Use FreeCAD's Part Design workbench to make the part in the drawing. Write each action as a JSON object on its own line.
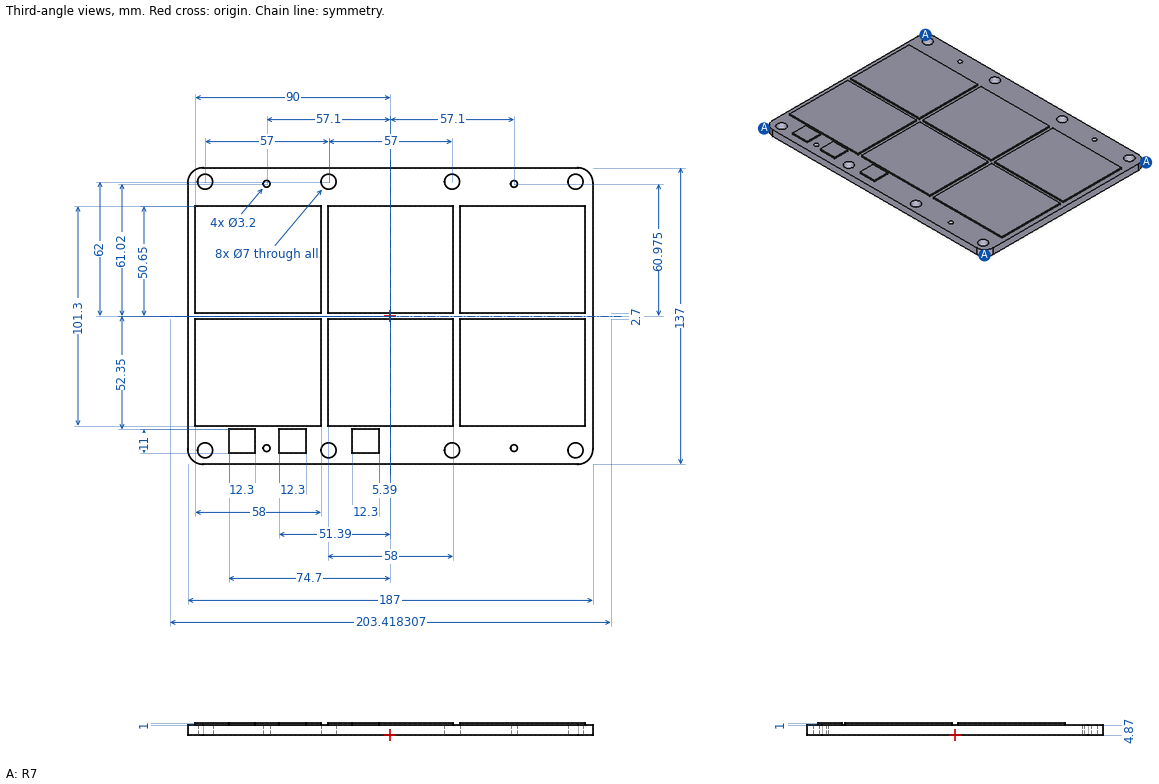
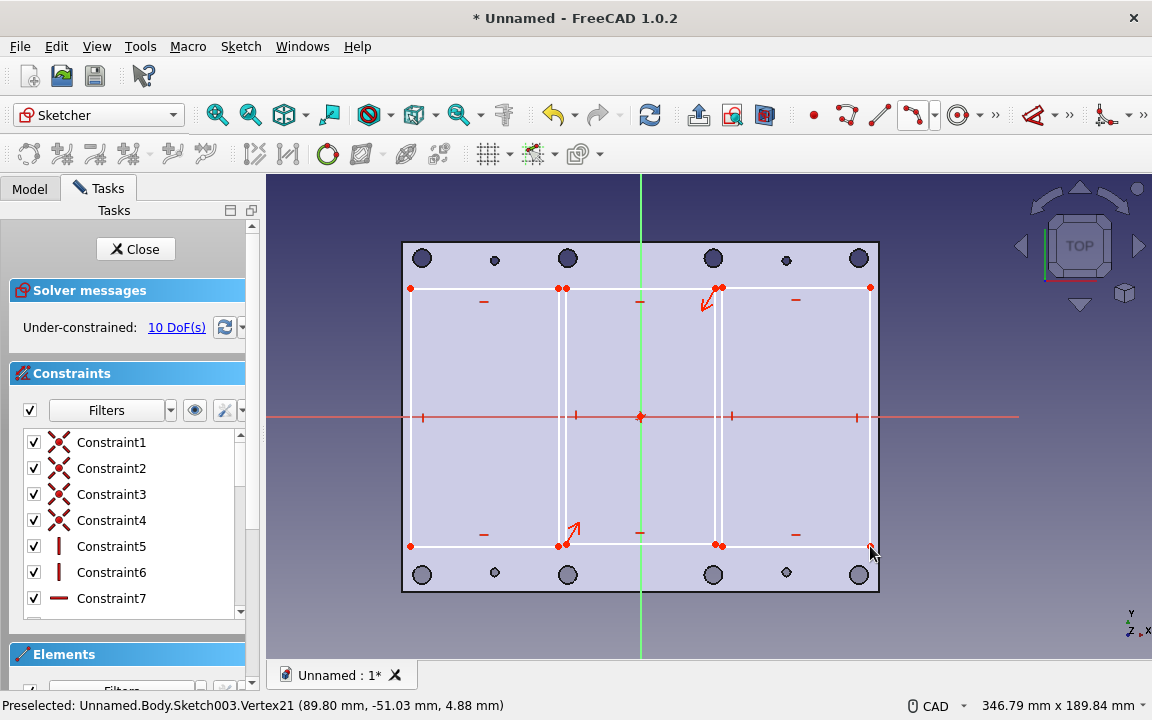
{"action": "scroll", "coordinate": [559, 289], "scroll_direction": "up", "scroll_amount": 3}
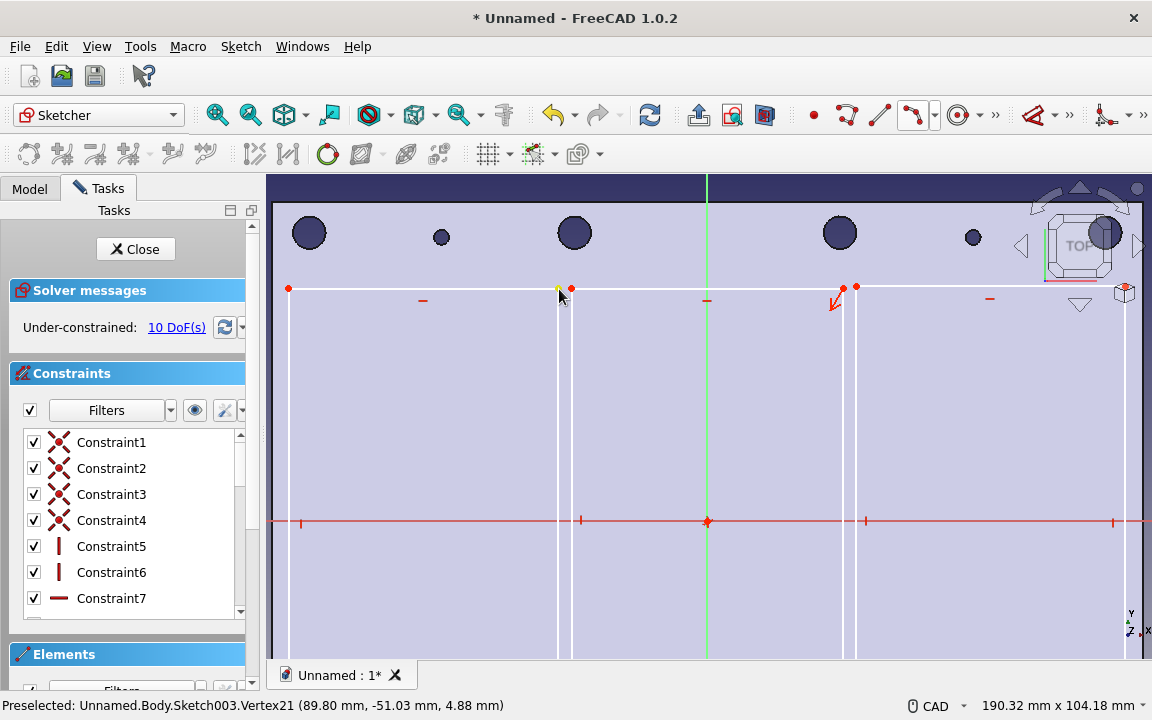
{"action": "left_click", "coordinate": [558, 289]}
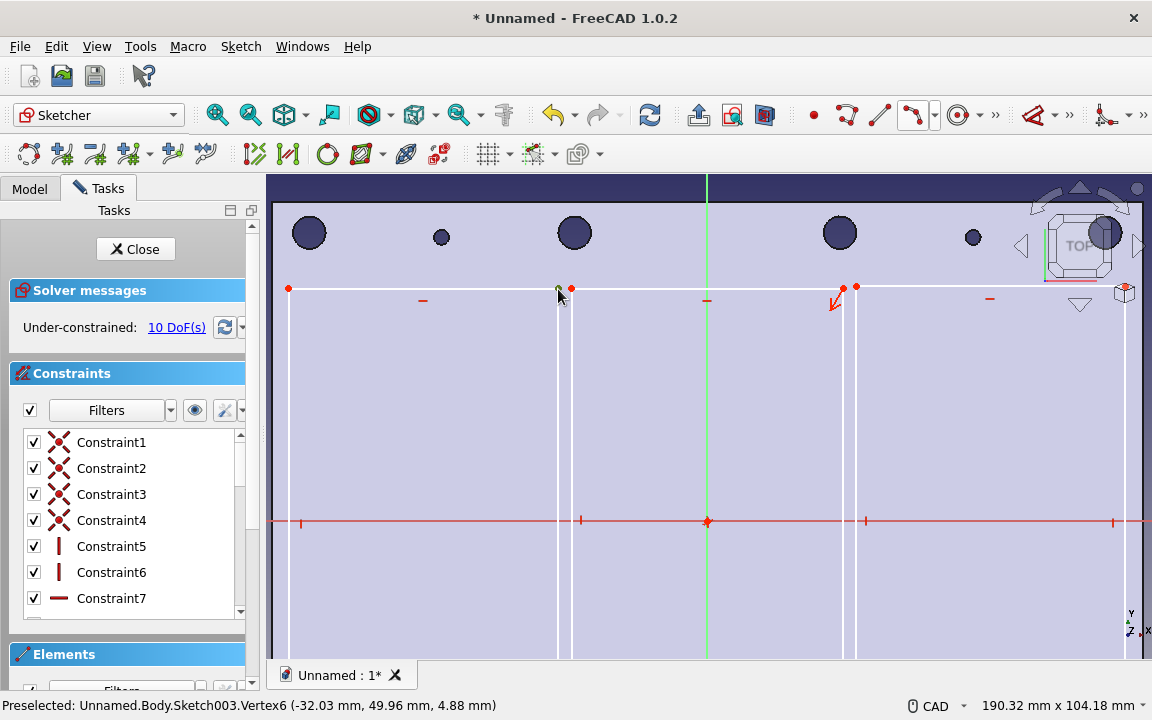
{"action": "left_click", "coordinate": [856, 286]}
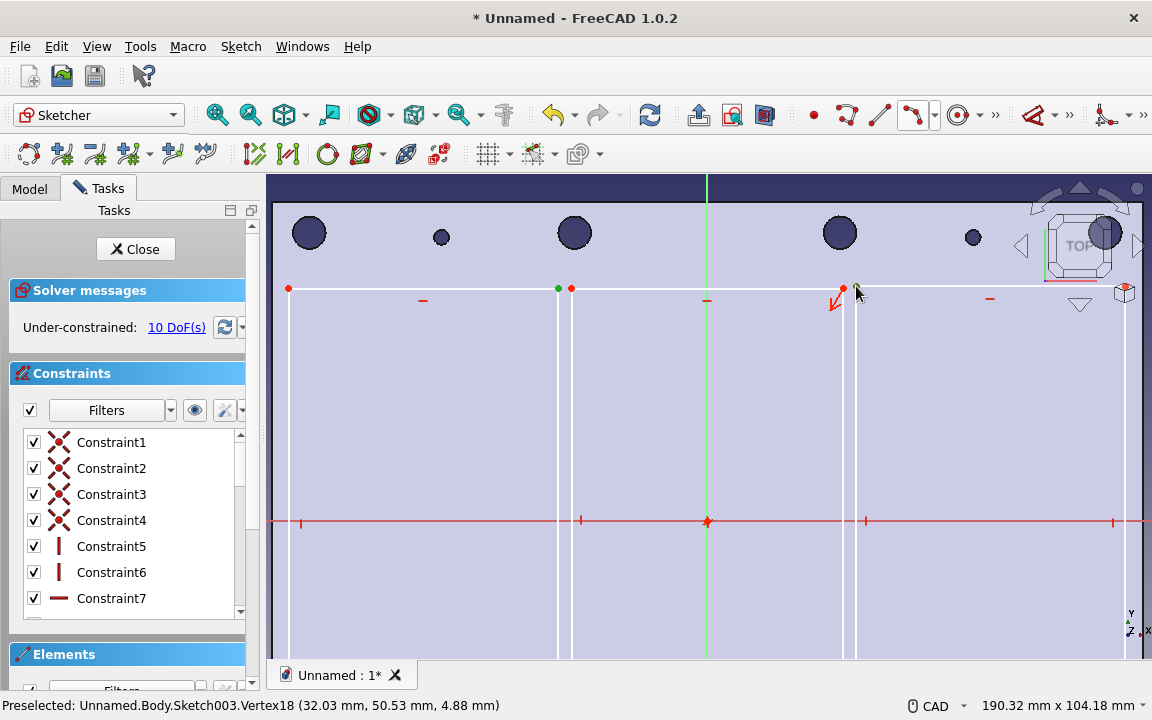
{"action": "left_click", "coordinate": [707, 600]}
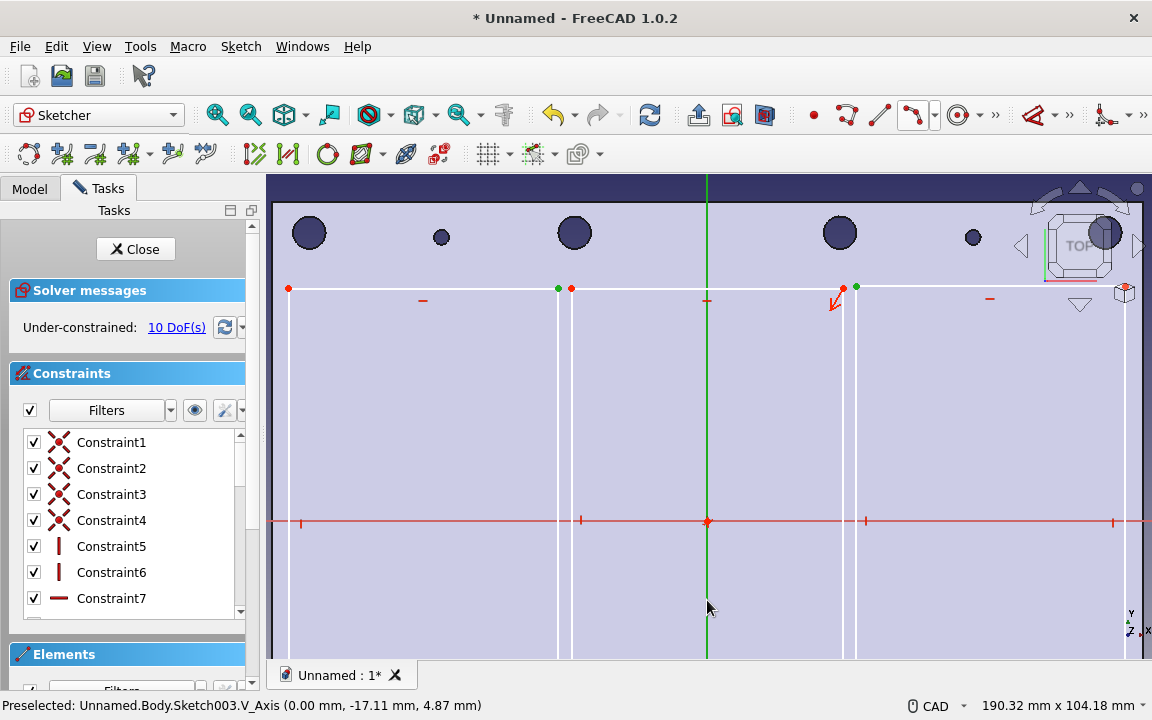
{"action": "key", "text": "s"}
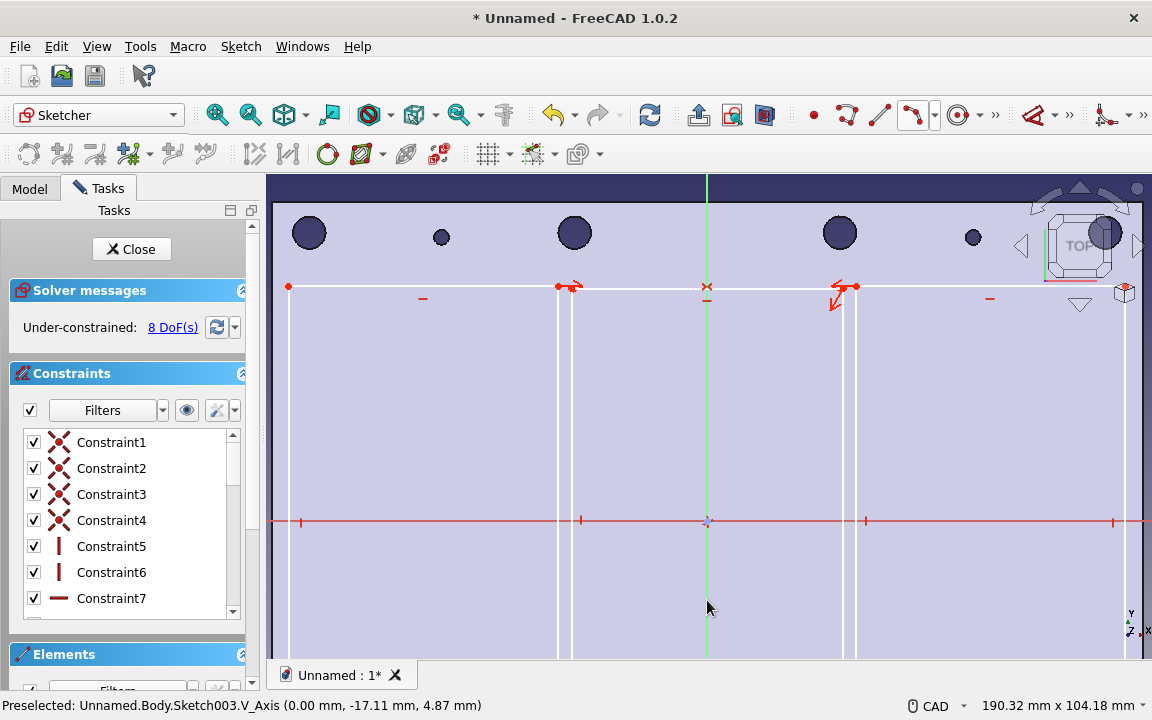
{"action": "scroll", "coordinate": [559, 289], "scroll_direction": "down", "scroll_amount": 3}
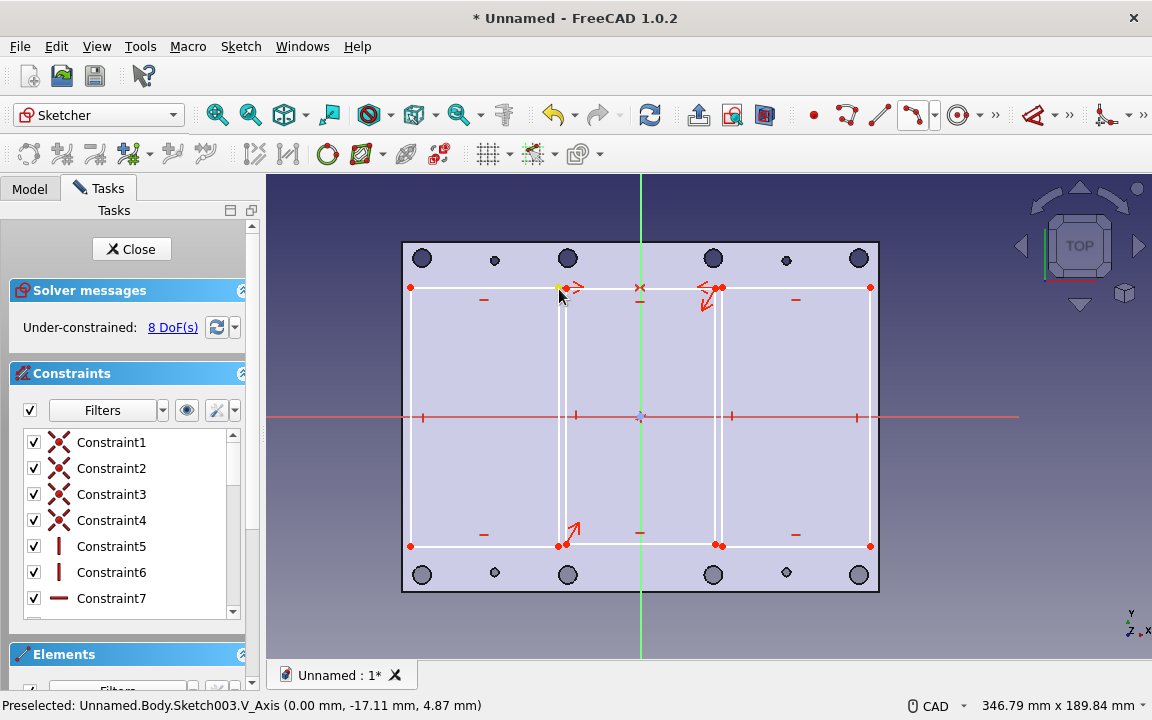
{"action": "left_click", "coordinate": [411, 547]}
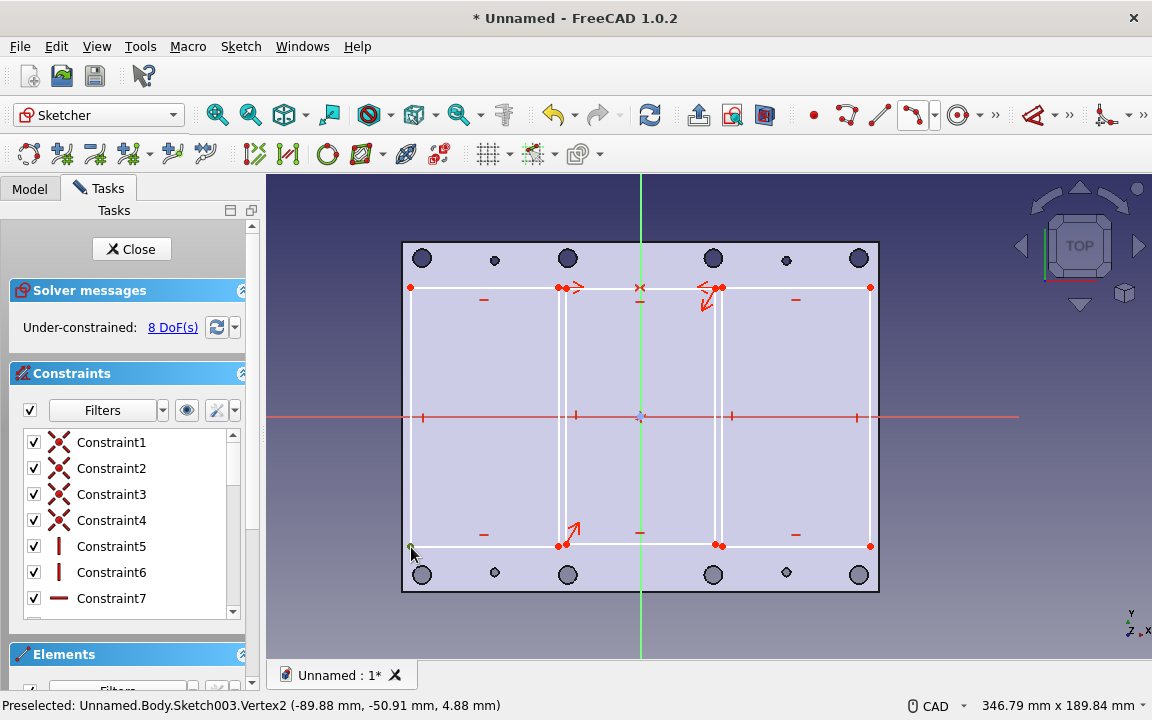
{"action": "left_click", "coordinate": [870, 547]}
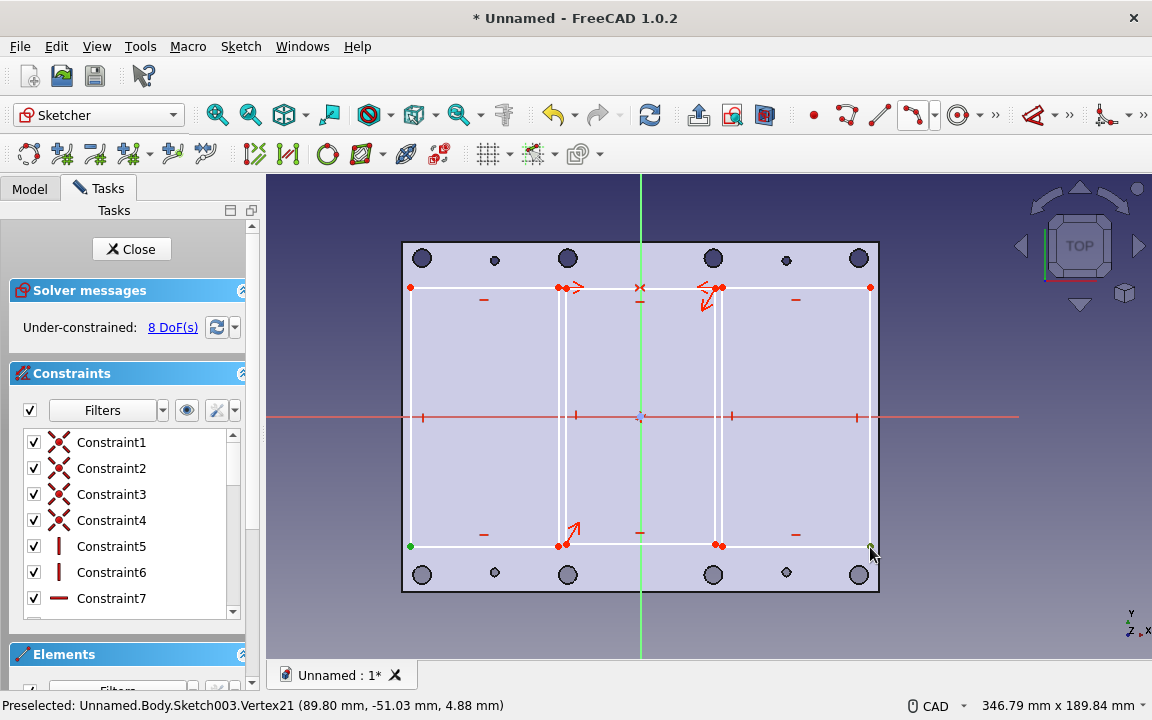
{"action": "left_click", "coordinate": [641, 600]}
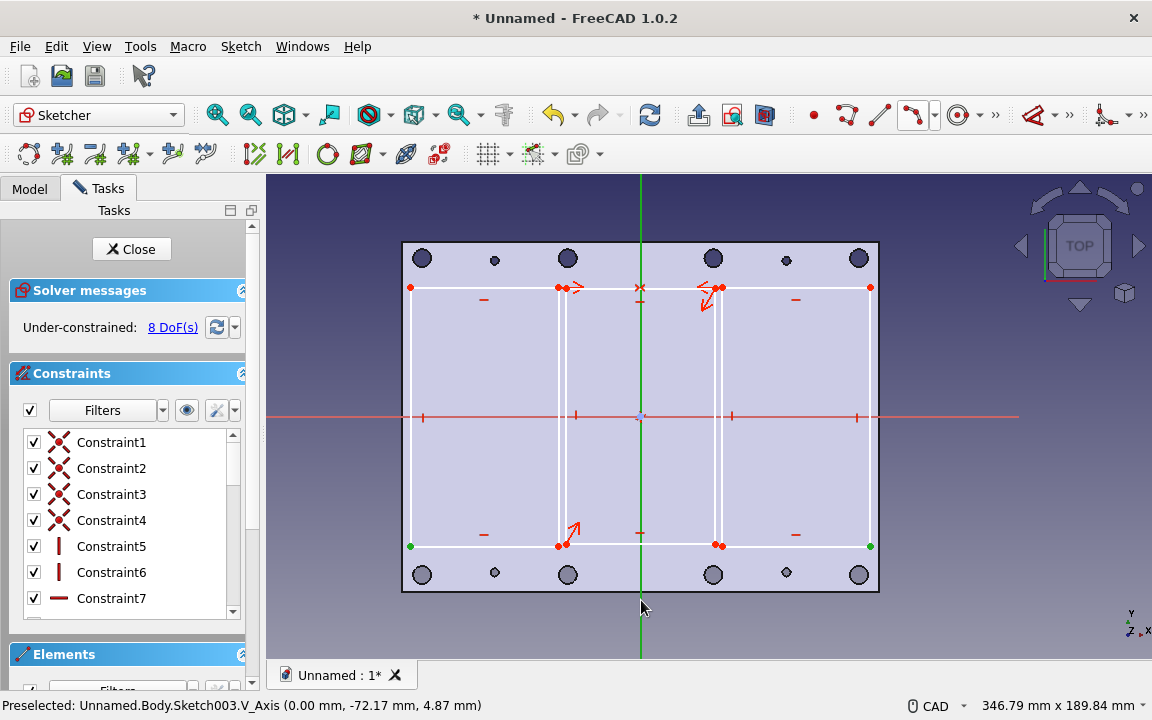
{"action": "key", "text": "s"}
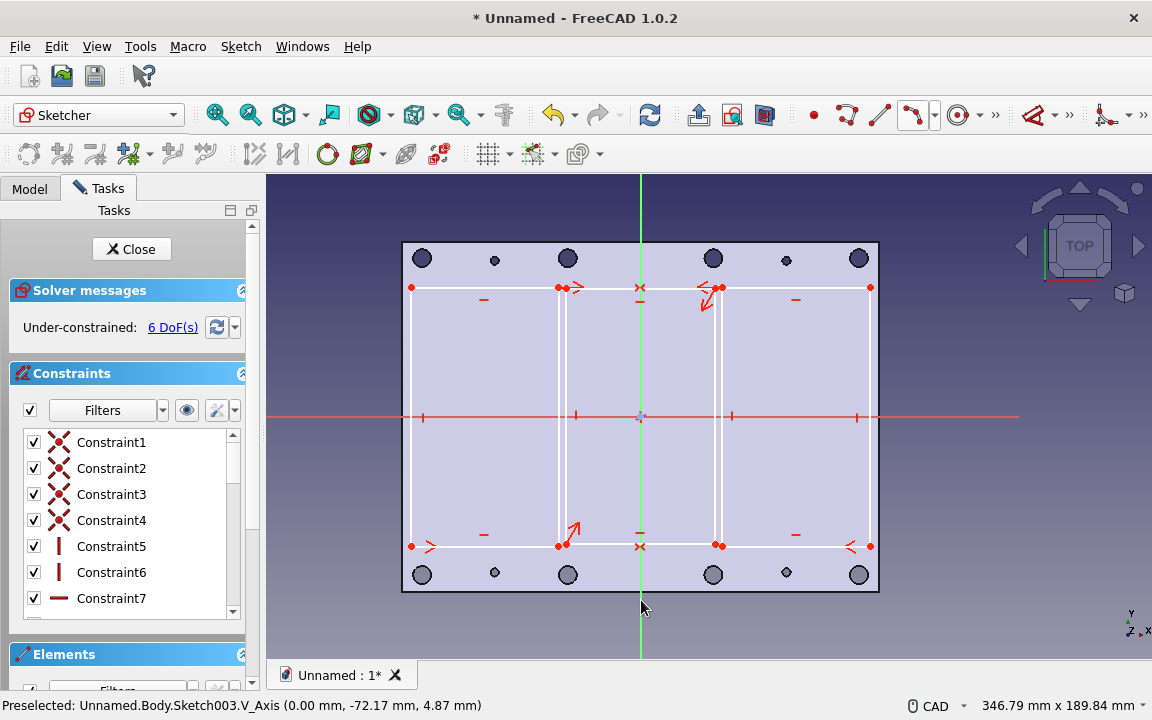
{"action": "key", "text": "d"}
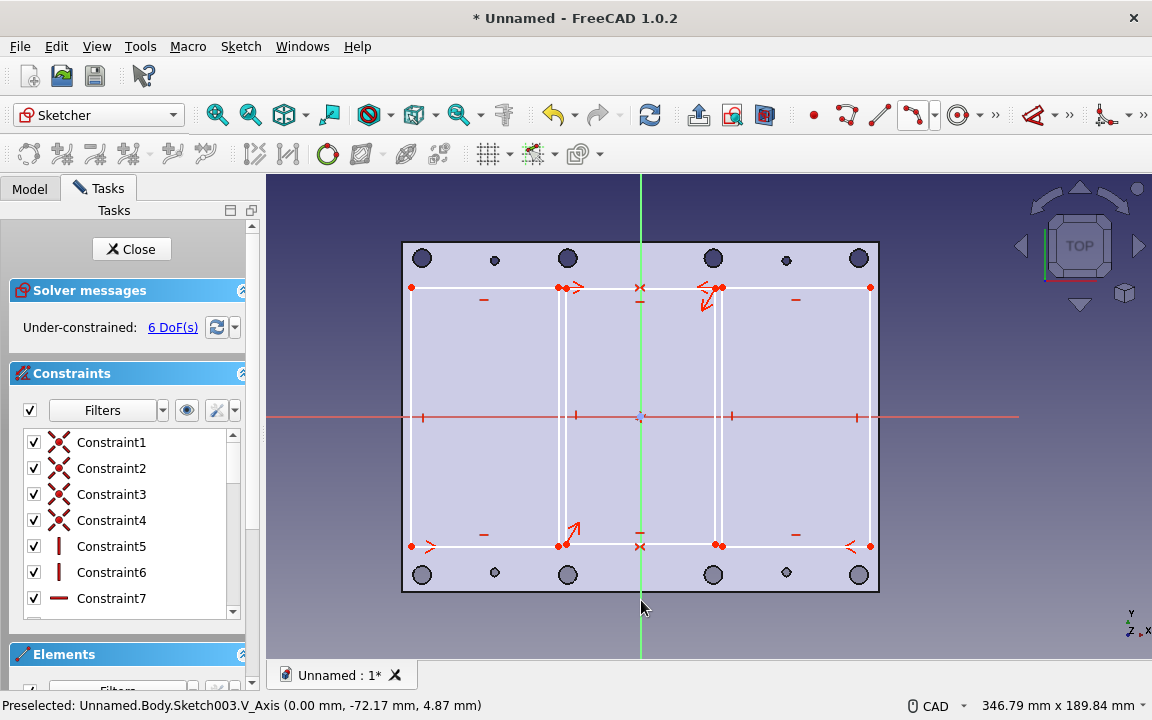
{"action": "left_click", "coordinate": [455, 547]}
{"action": "left_click", "coordinate": [485, 581]}